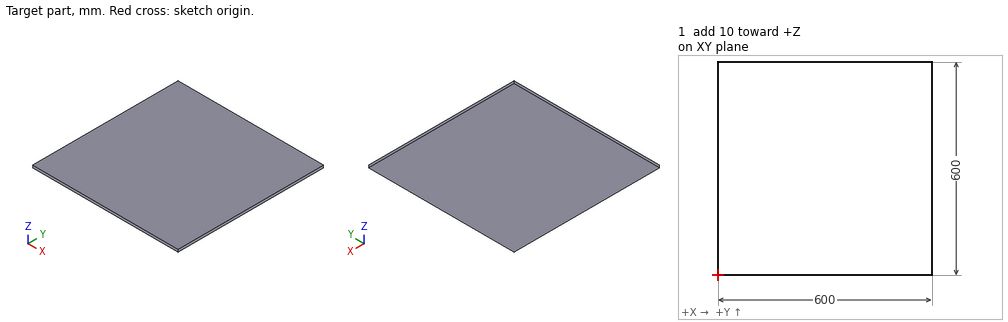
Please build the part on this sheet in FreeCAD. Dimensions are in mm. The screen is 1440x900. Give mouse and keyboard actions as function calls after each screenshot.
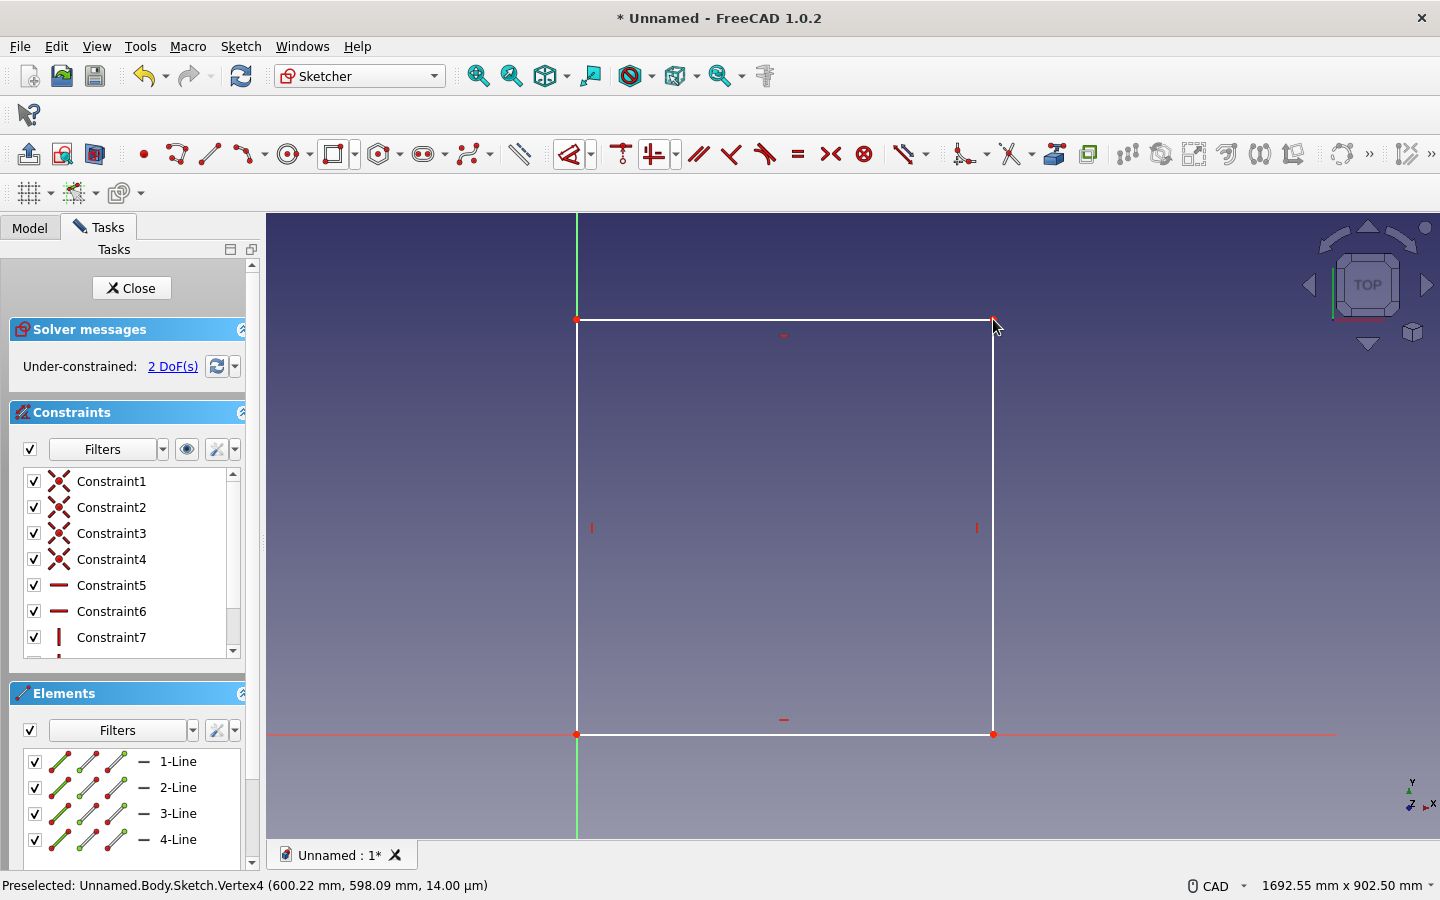
click(568, 154)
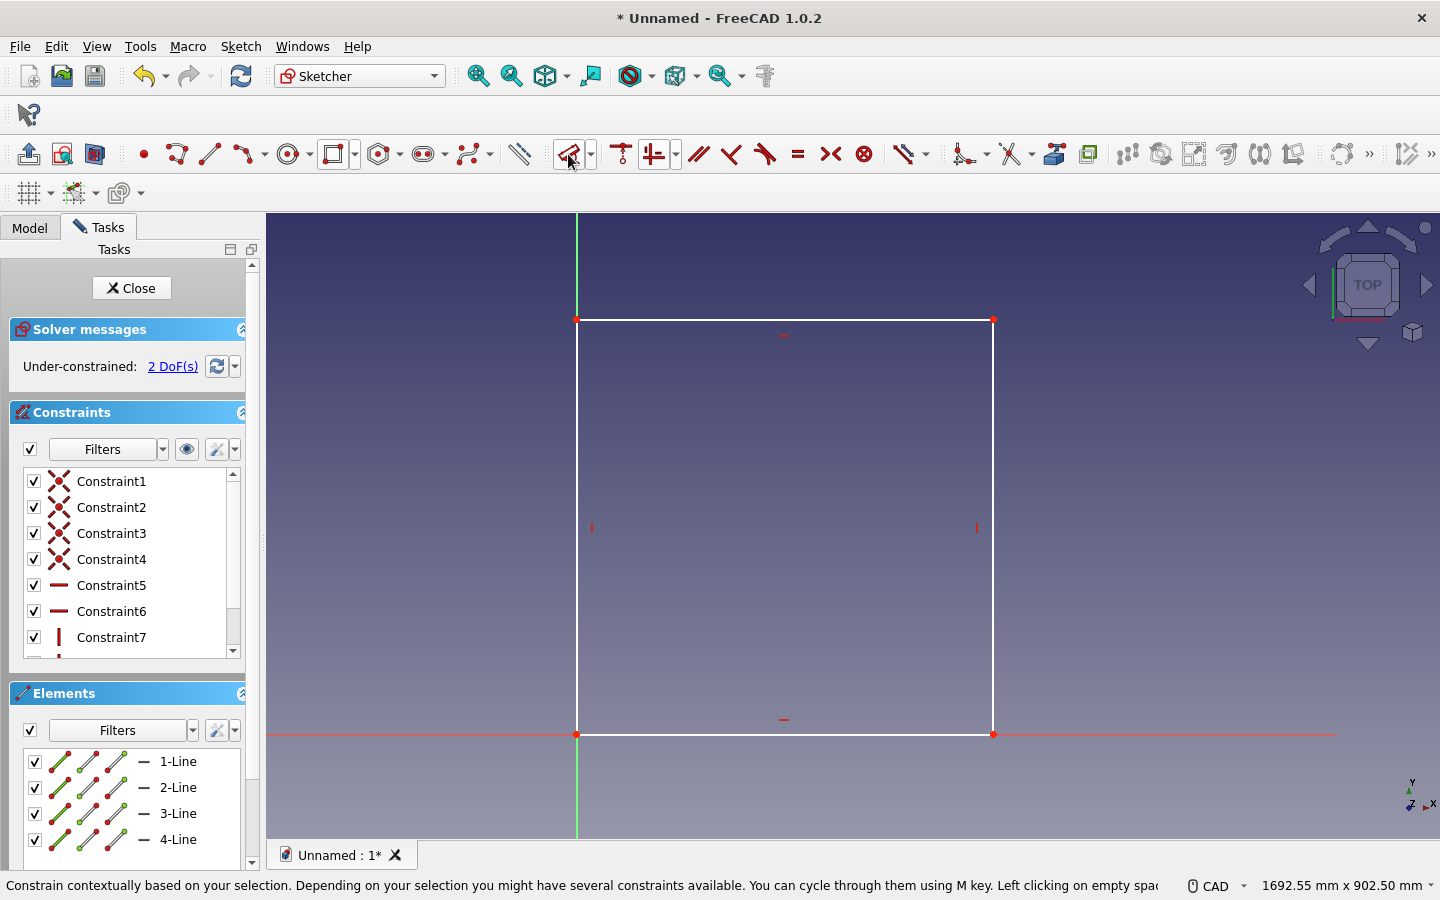
click(702, 735)
click(785, 769)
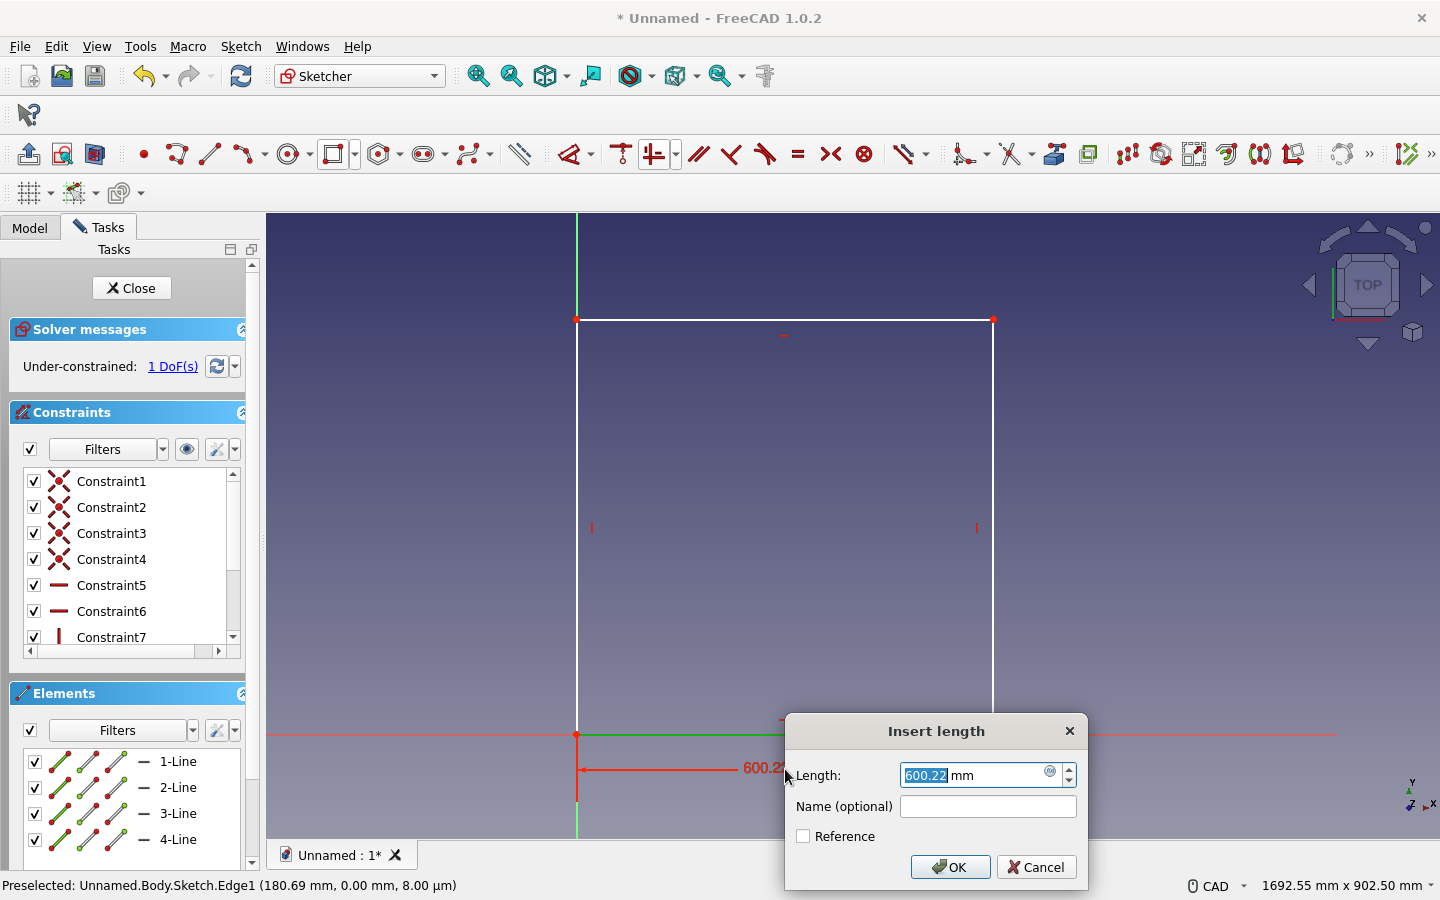
text(600)
key(Return)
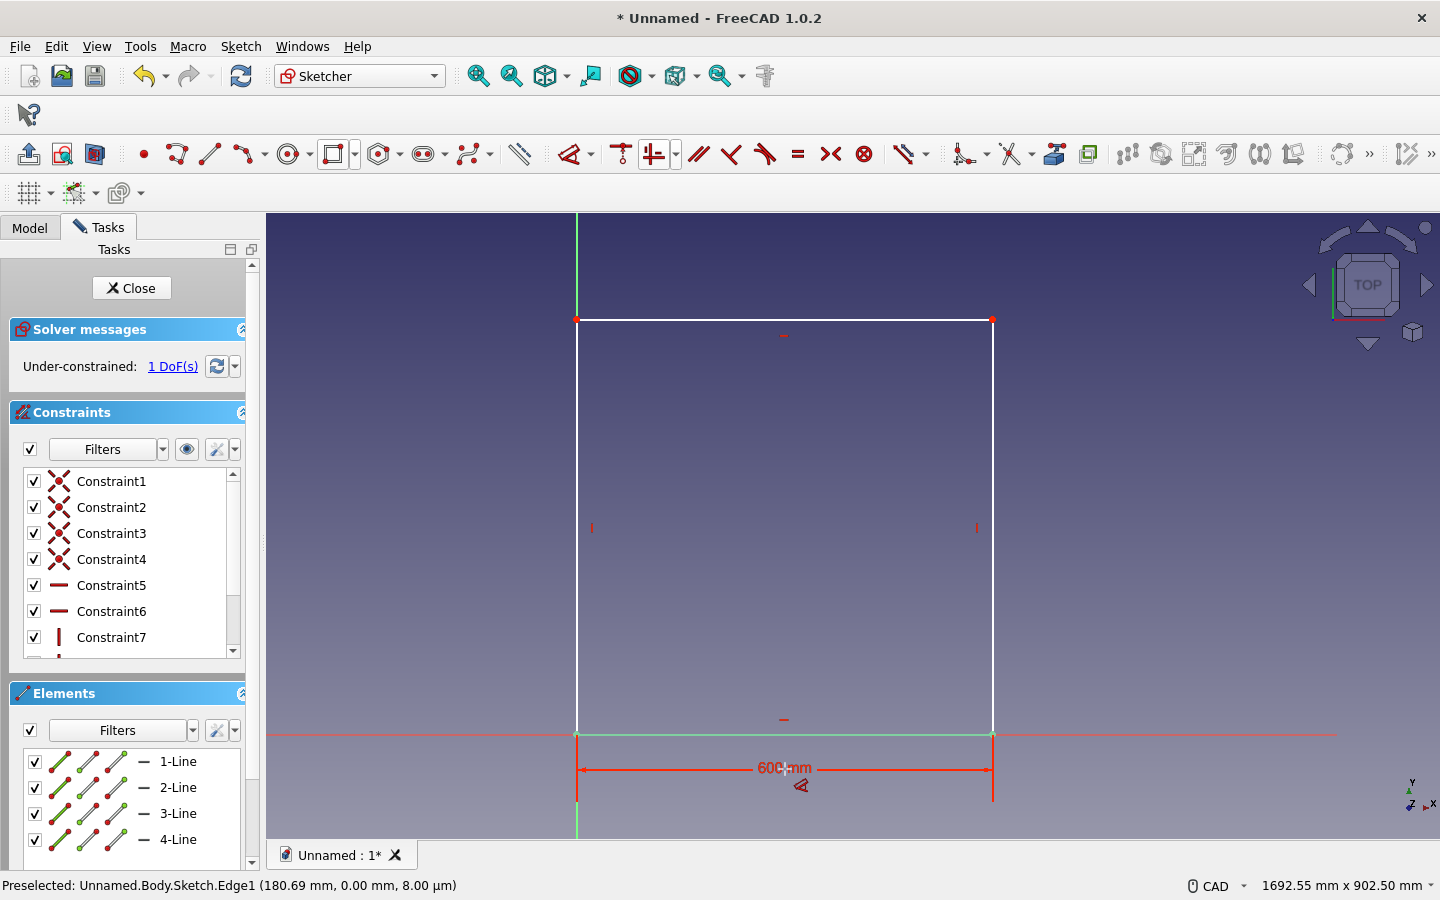
click(993, 610)
click(1027, 527)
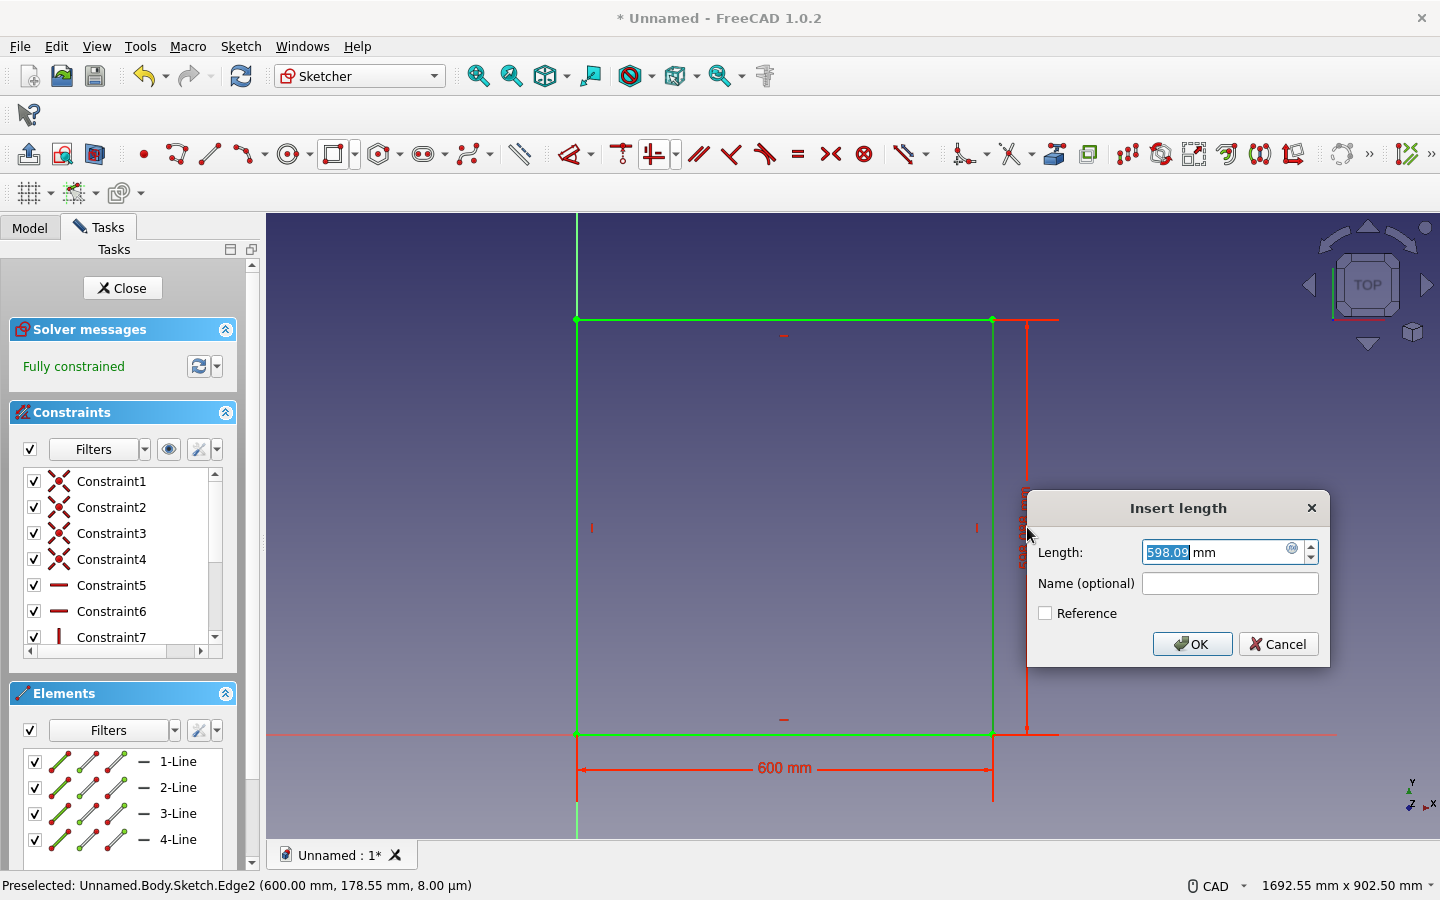
text(600)
key(Return)
key(Escape)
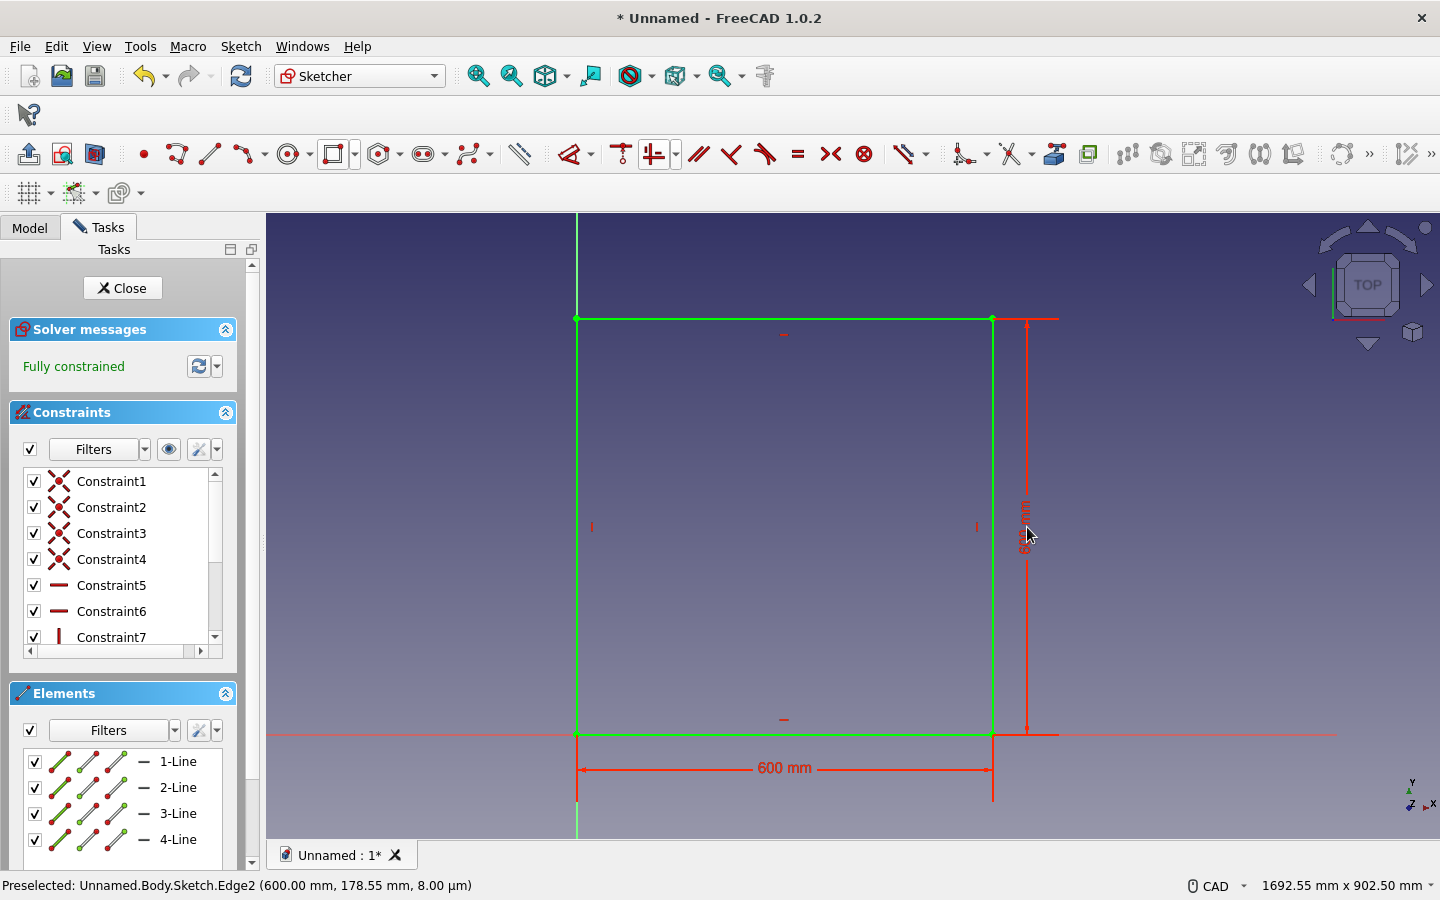
click(123, 288)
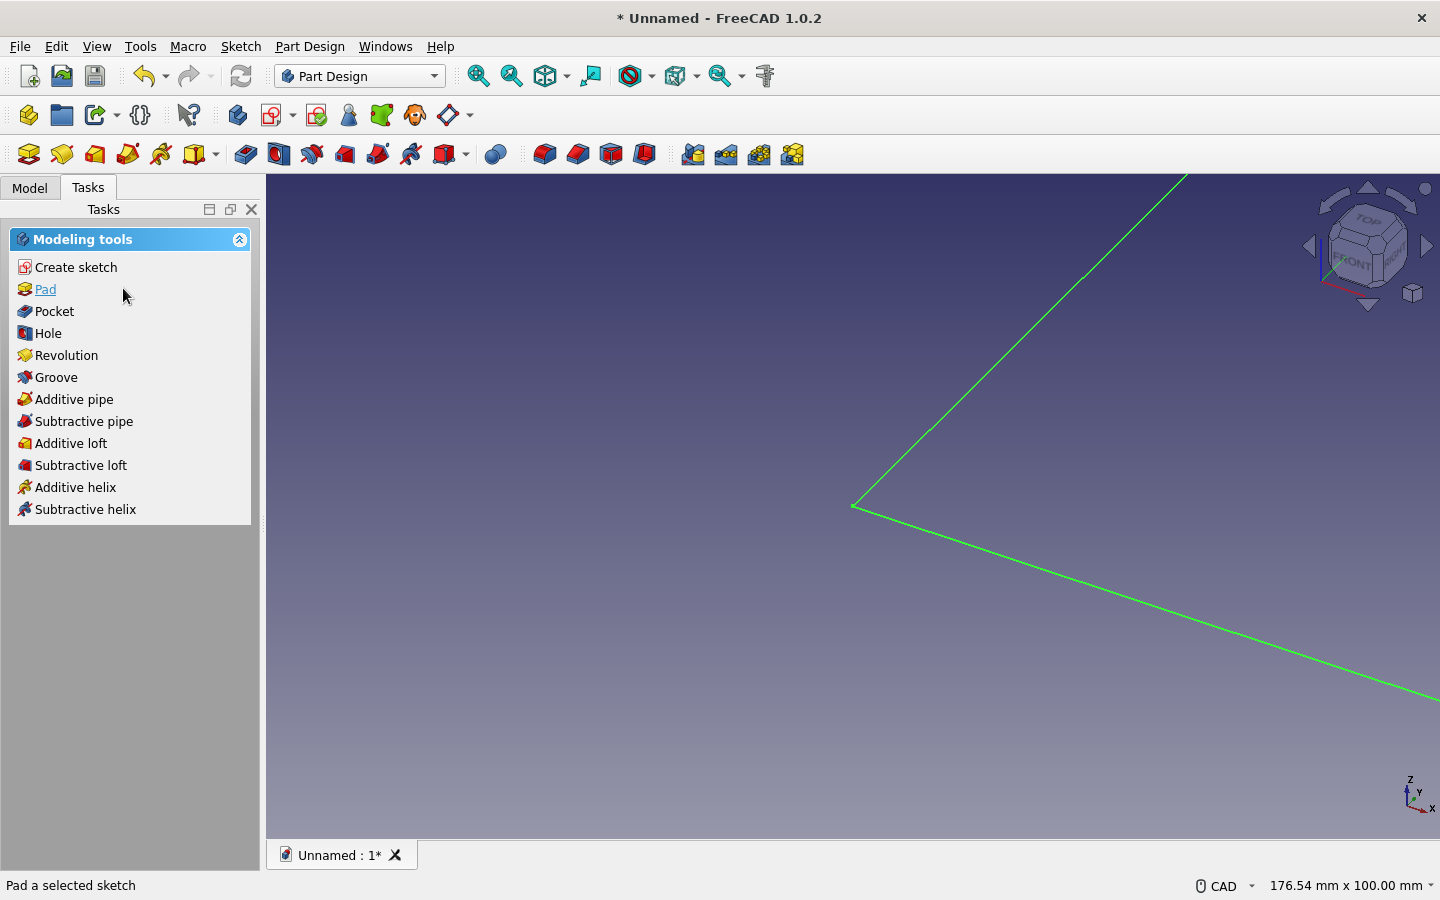
click(29, 154)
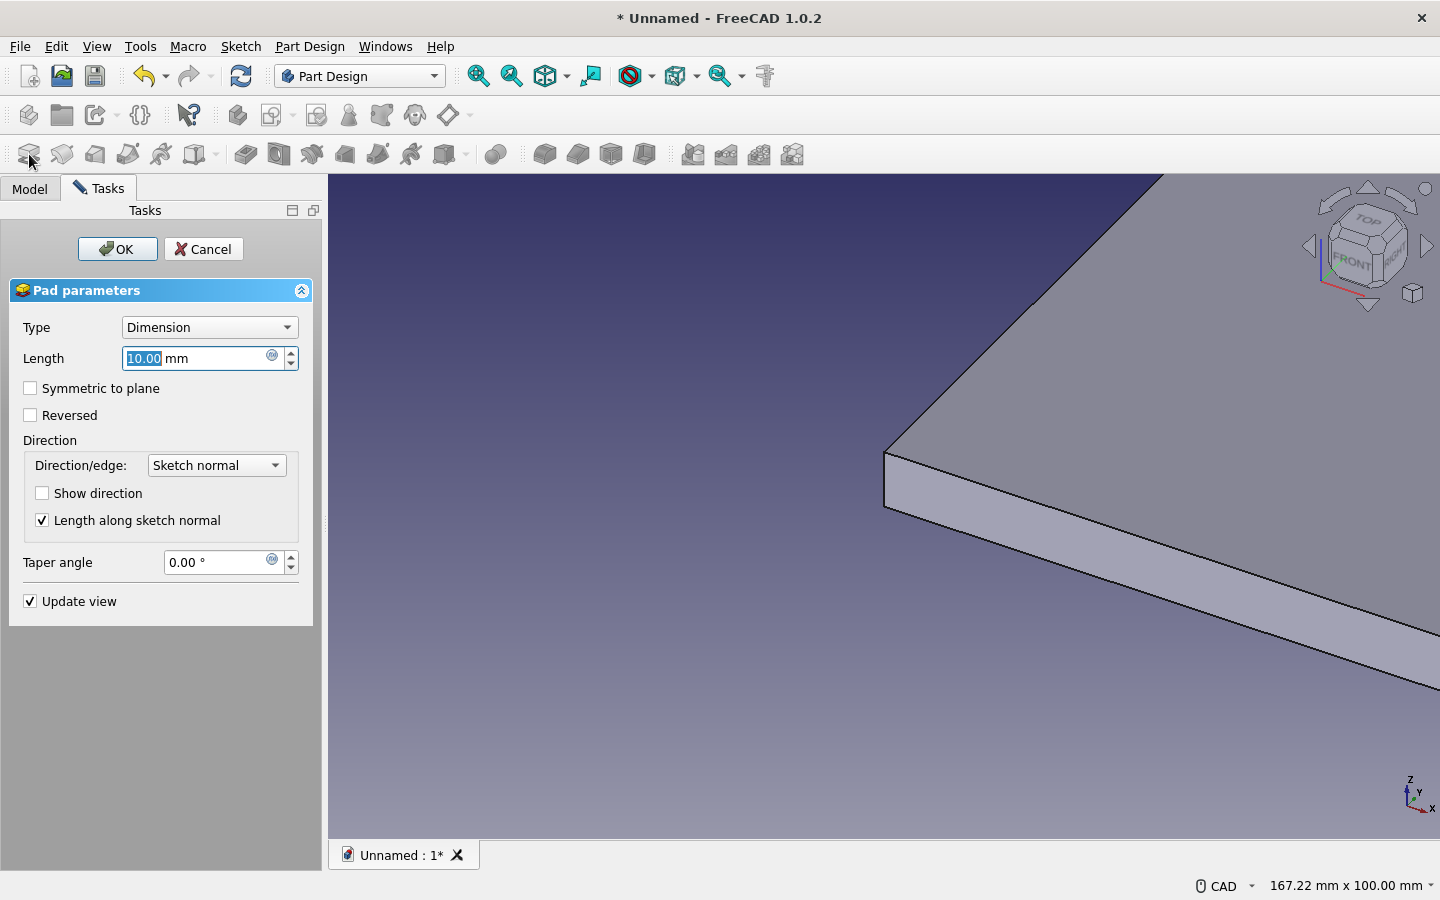
text(10)
key(Tab)